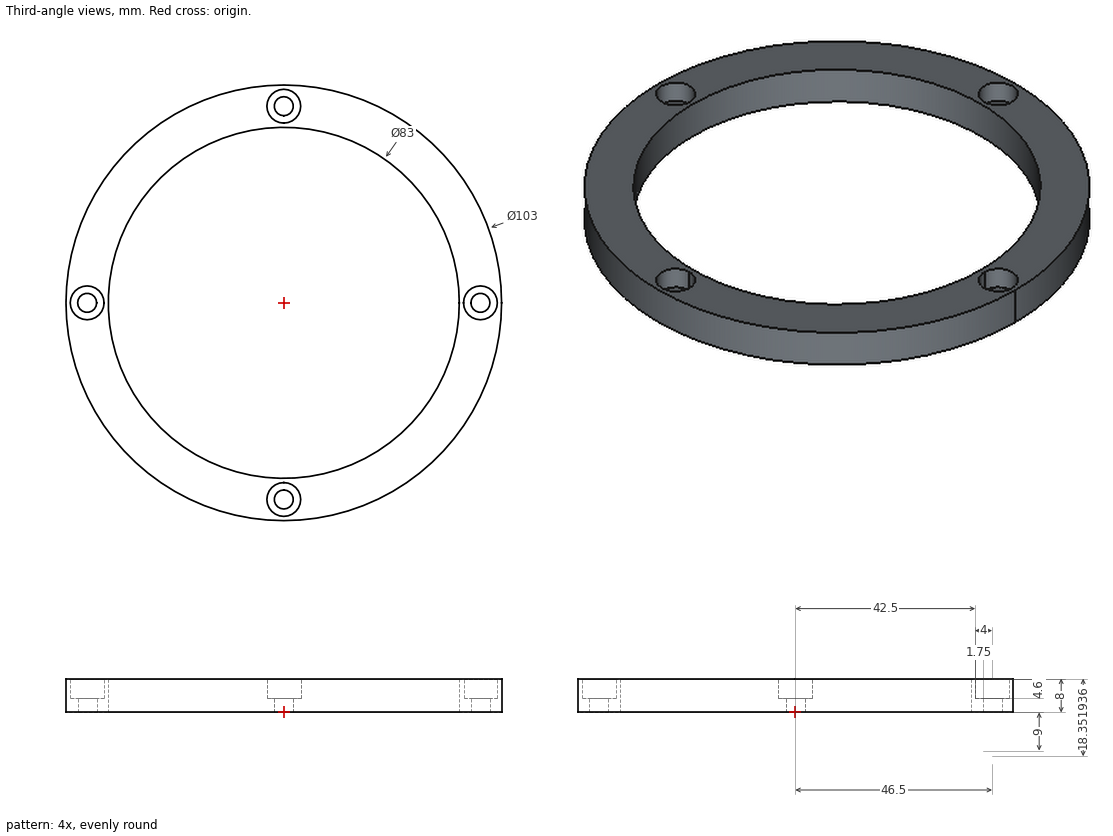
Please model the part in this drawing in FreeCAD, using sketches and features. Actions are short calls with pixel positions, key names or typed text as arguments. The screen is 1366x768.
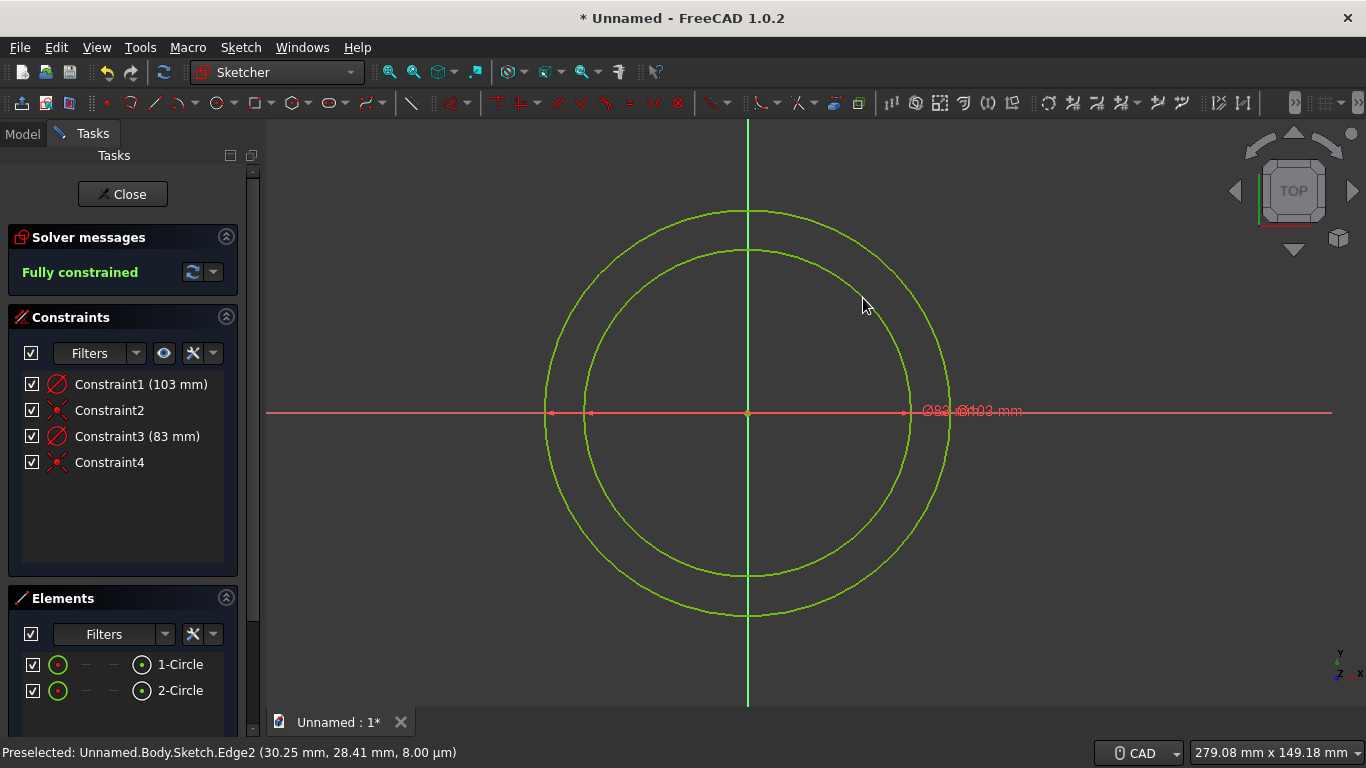
click(123, 194)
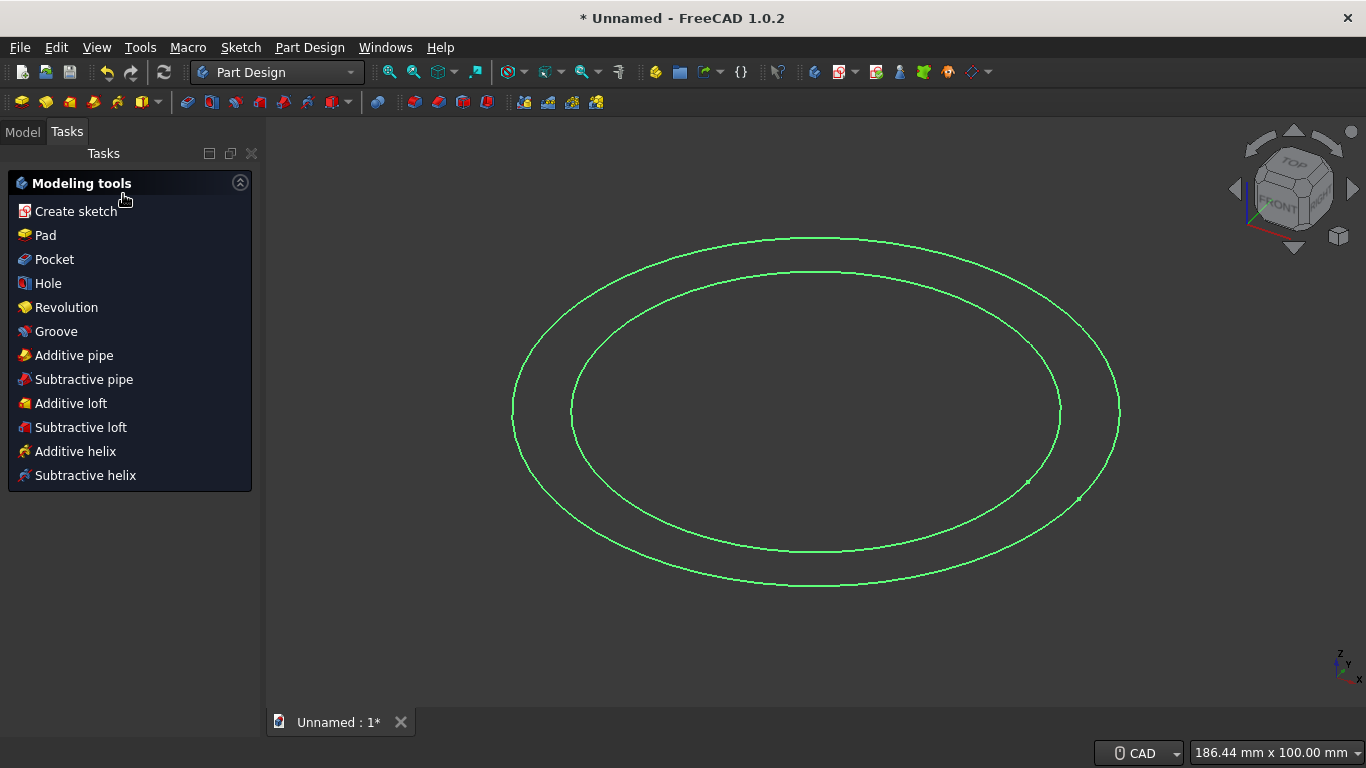
click(22, 102)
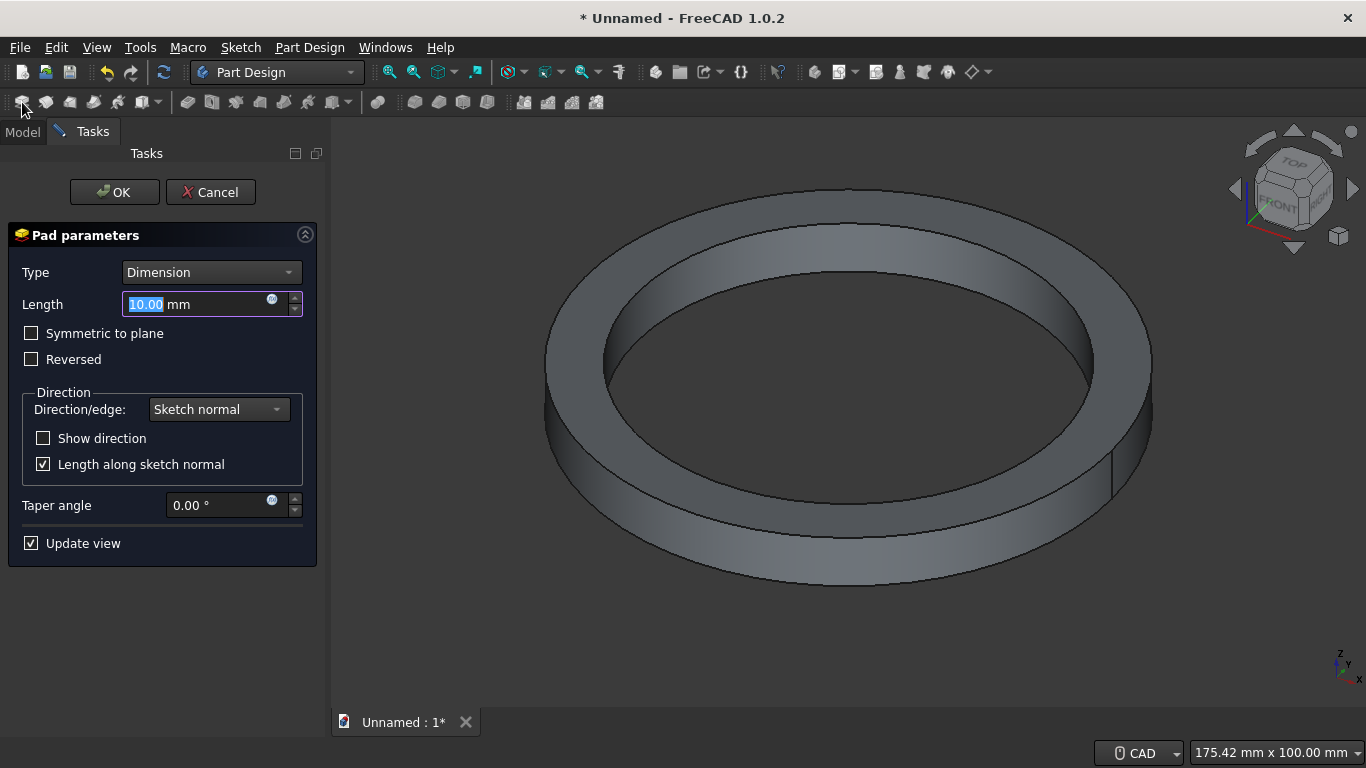
text(8)
key(Tab)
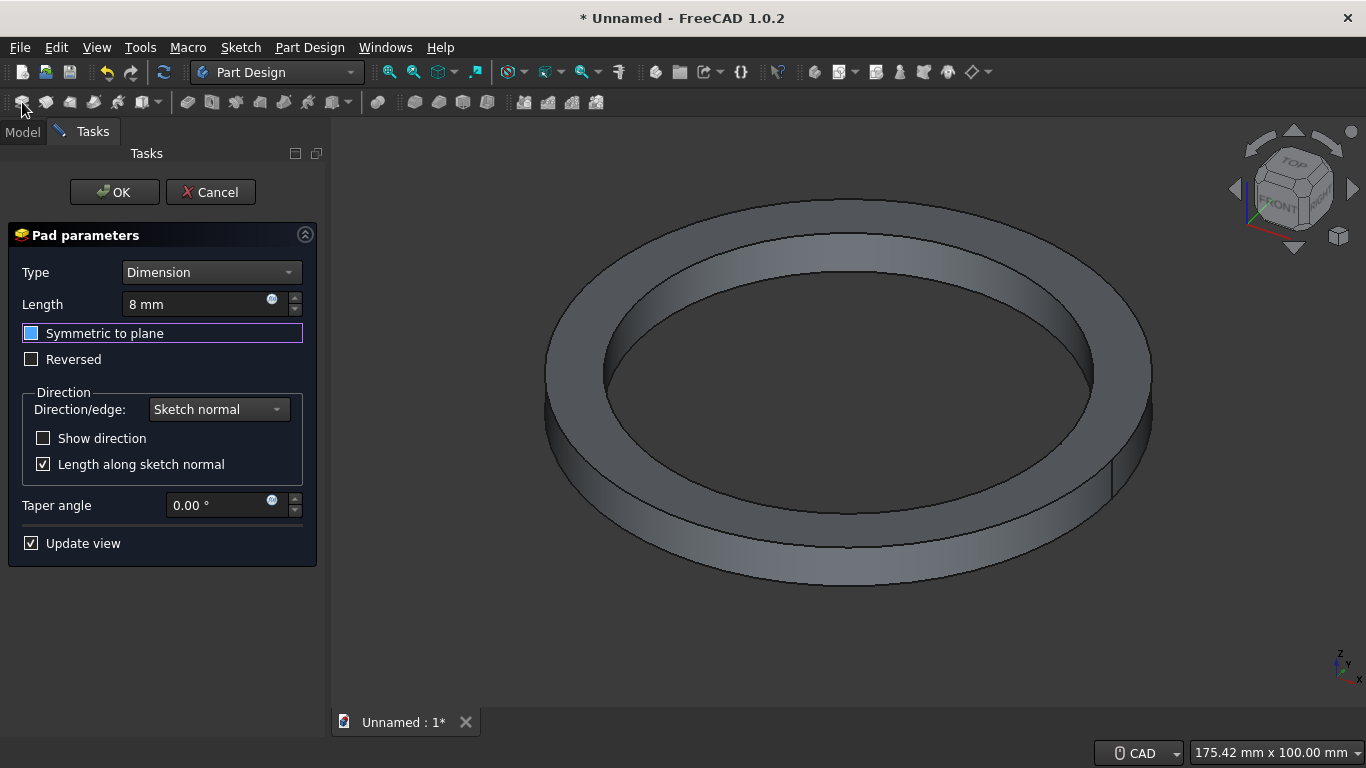
click(115, 192)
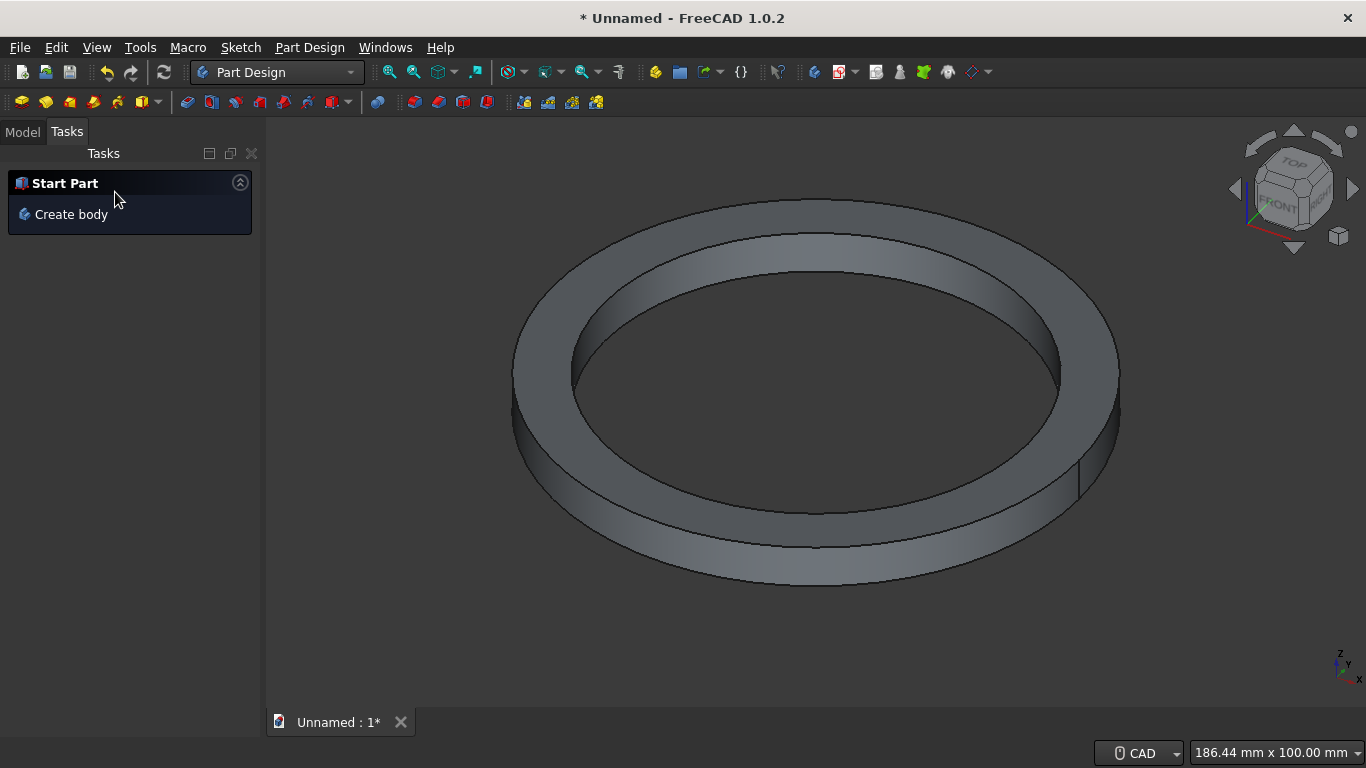
click(840, 72)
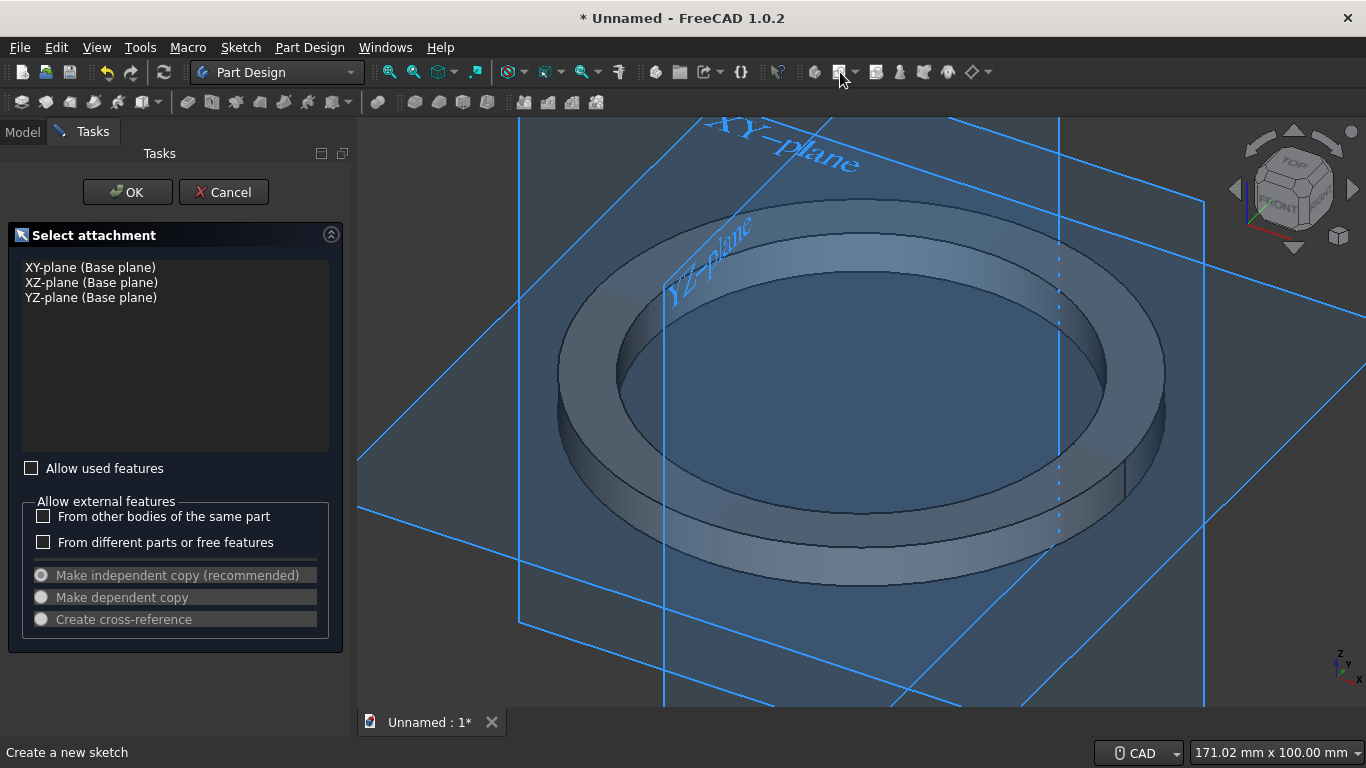
click(82, 298)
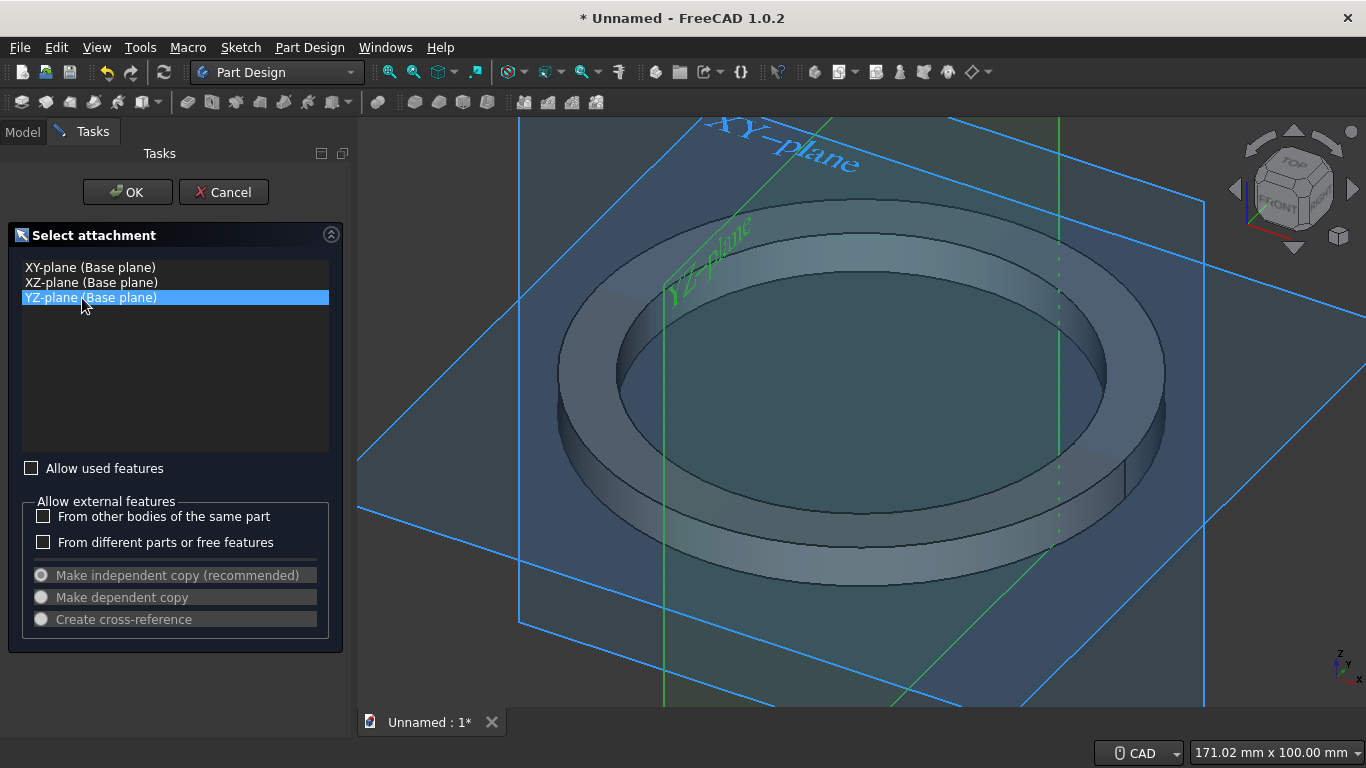
click(128, 192)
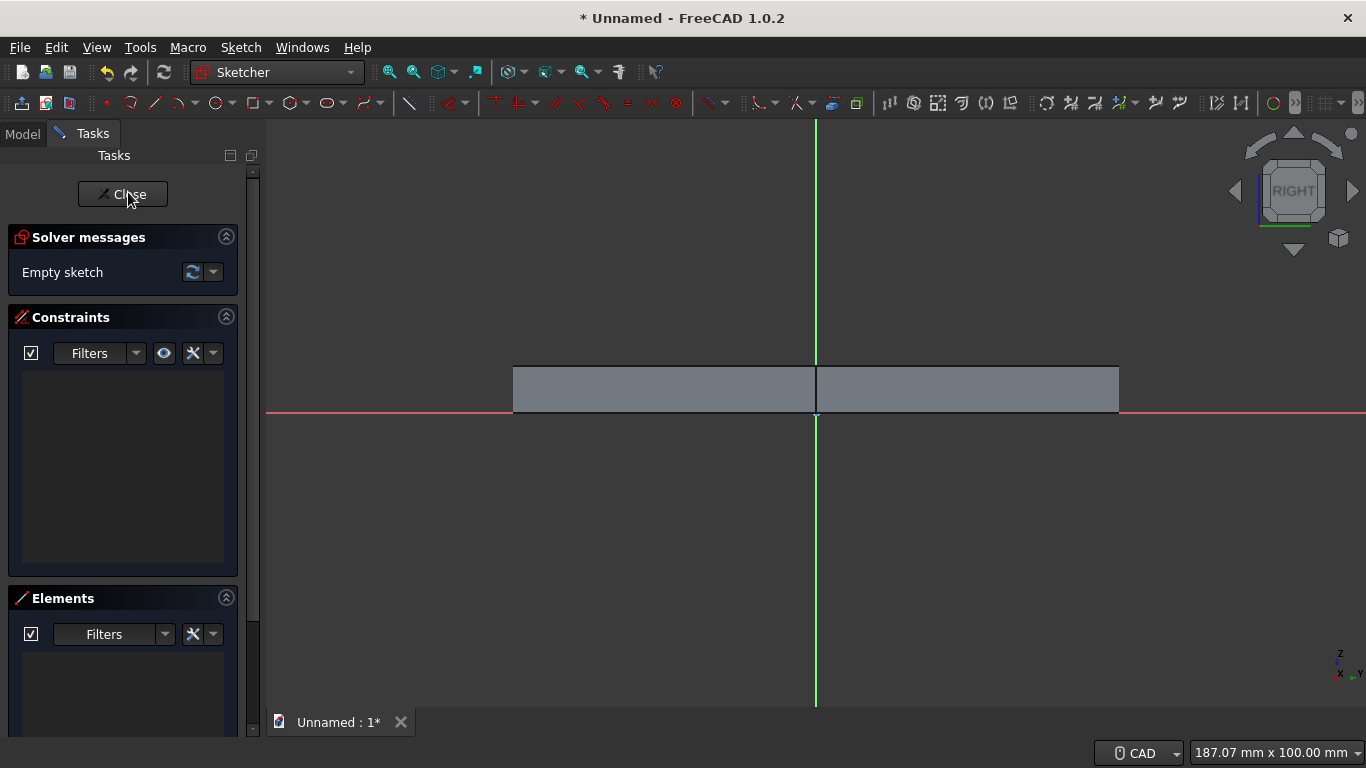
key(q)
key(s)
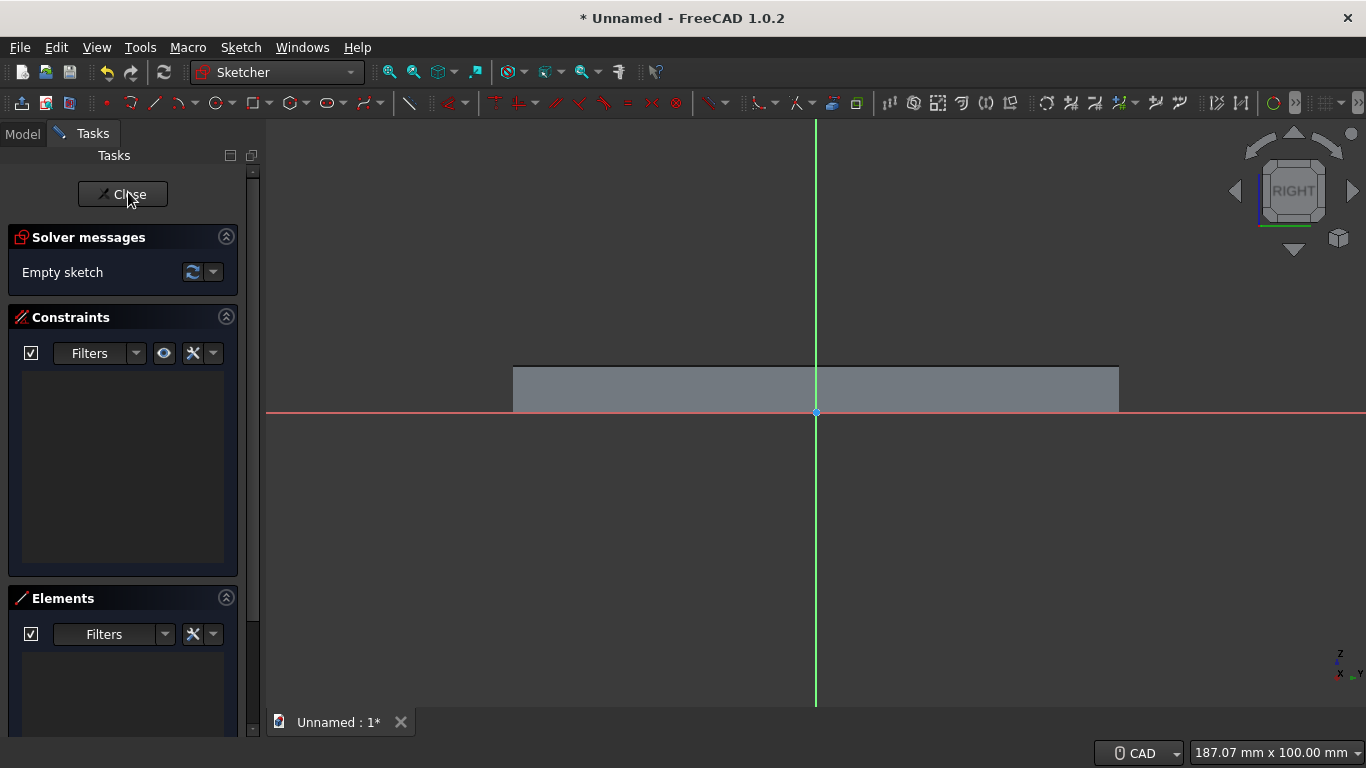
scroll(1120, 465, up, 4)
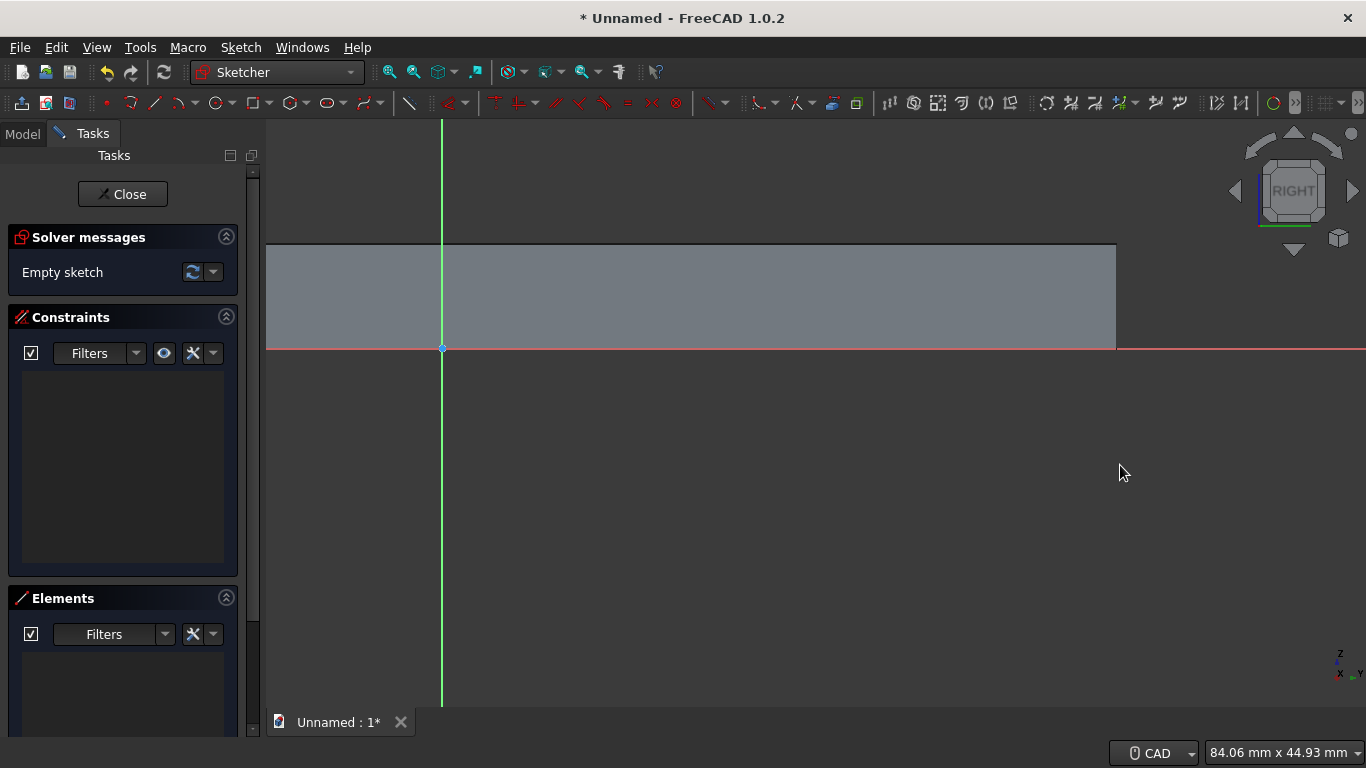
key(g)
key(m)